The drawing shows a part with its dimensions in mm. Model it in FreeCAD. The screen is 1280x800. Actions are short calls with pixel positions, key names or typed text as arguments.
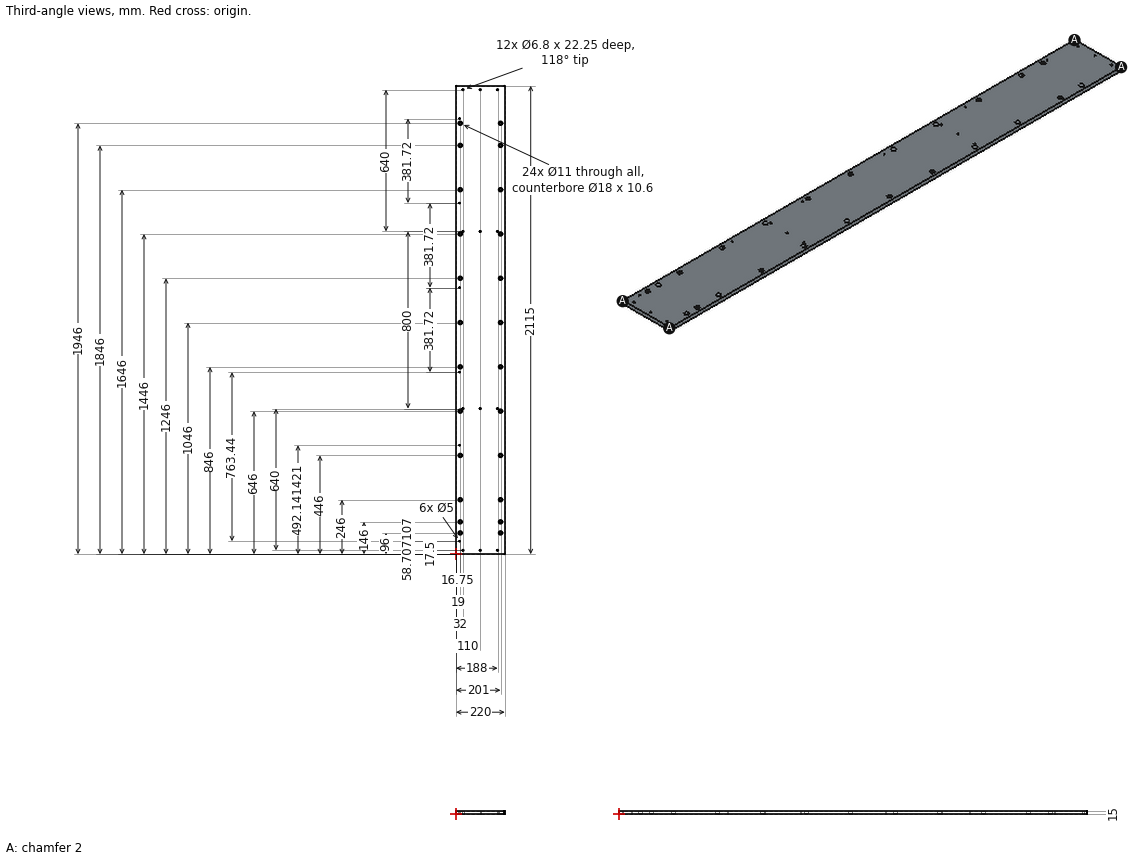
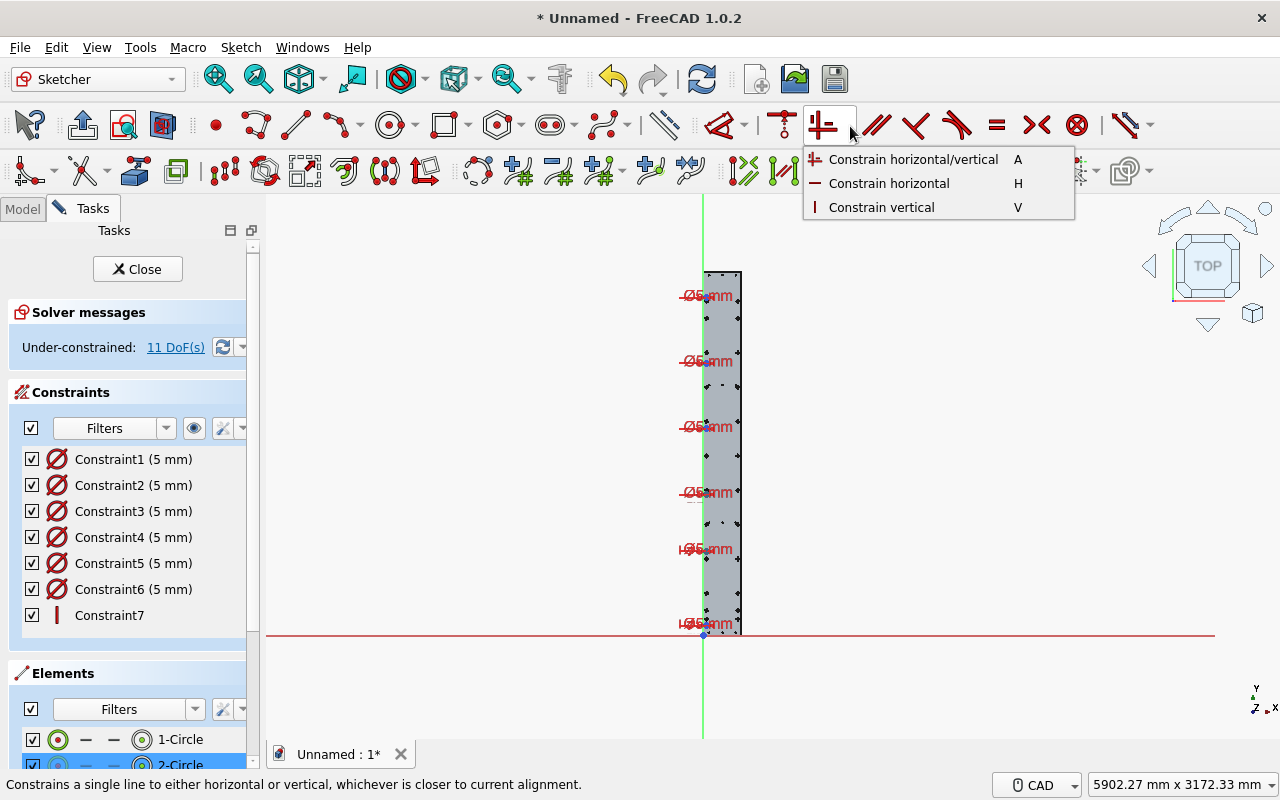
click(939, 207)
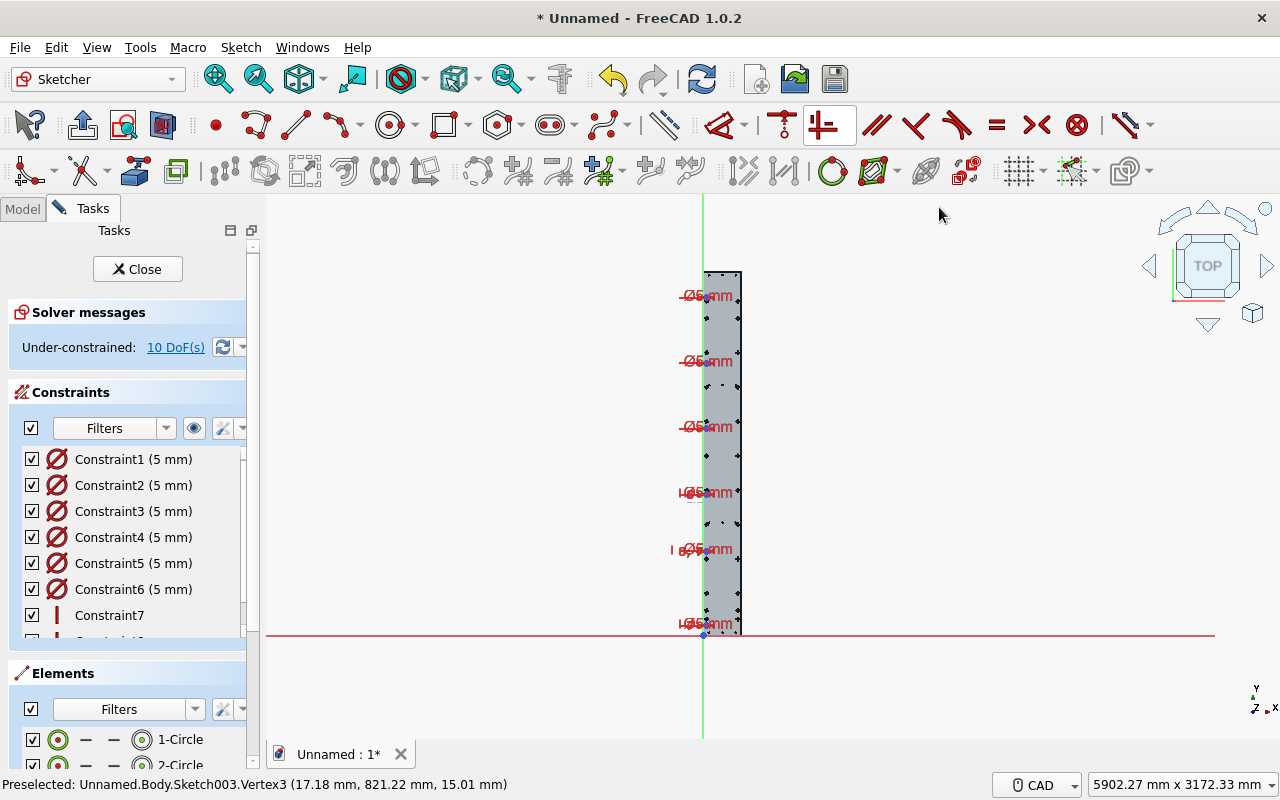
click(706, 495)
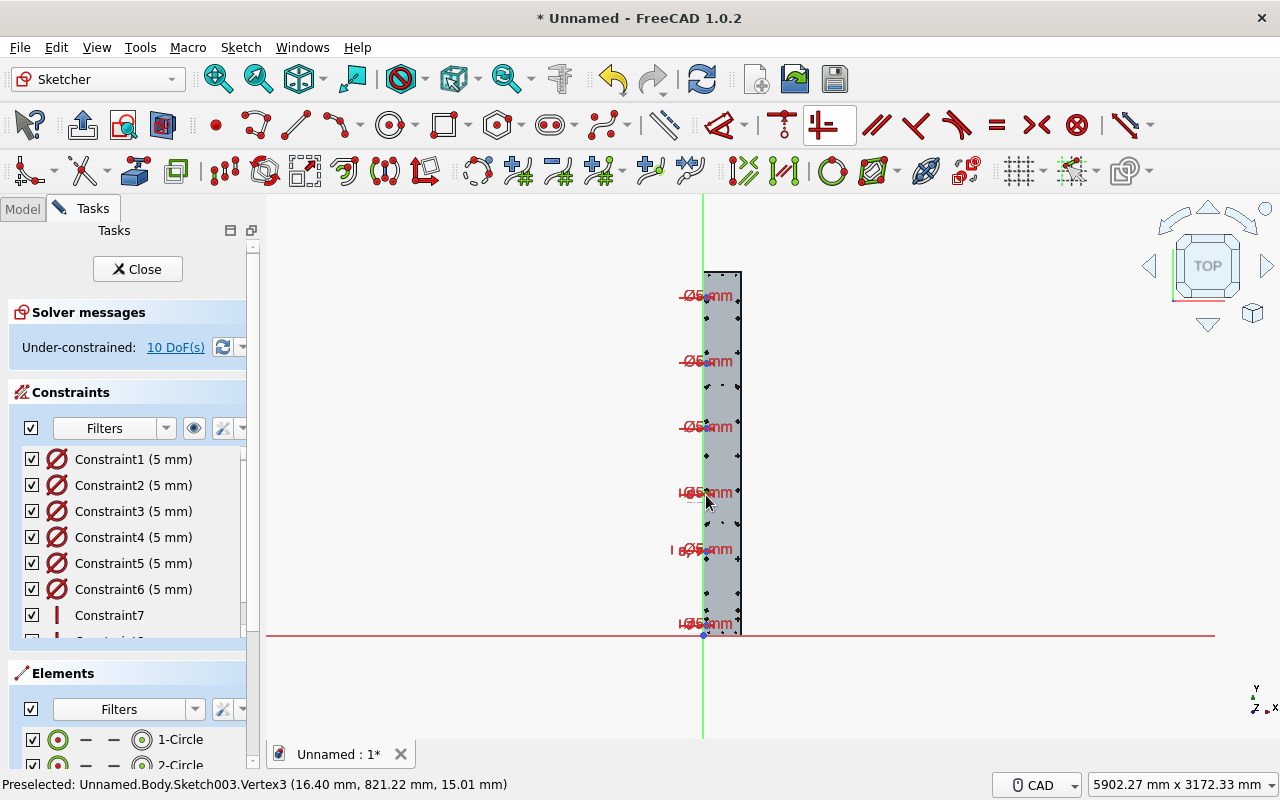
click(706, 429)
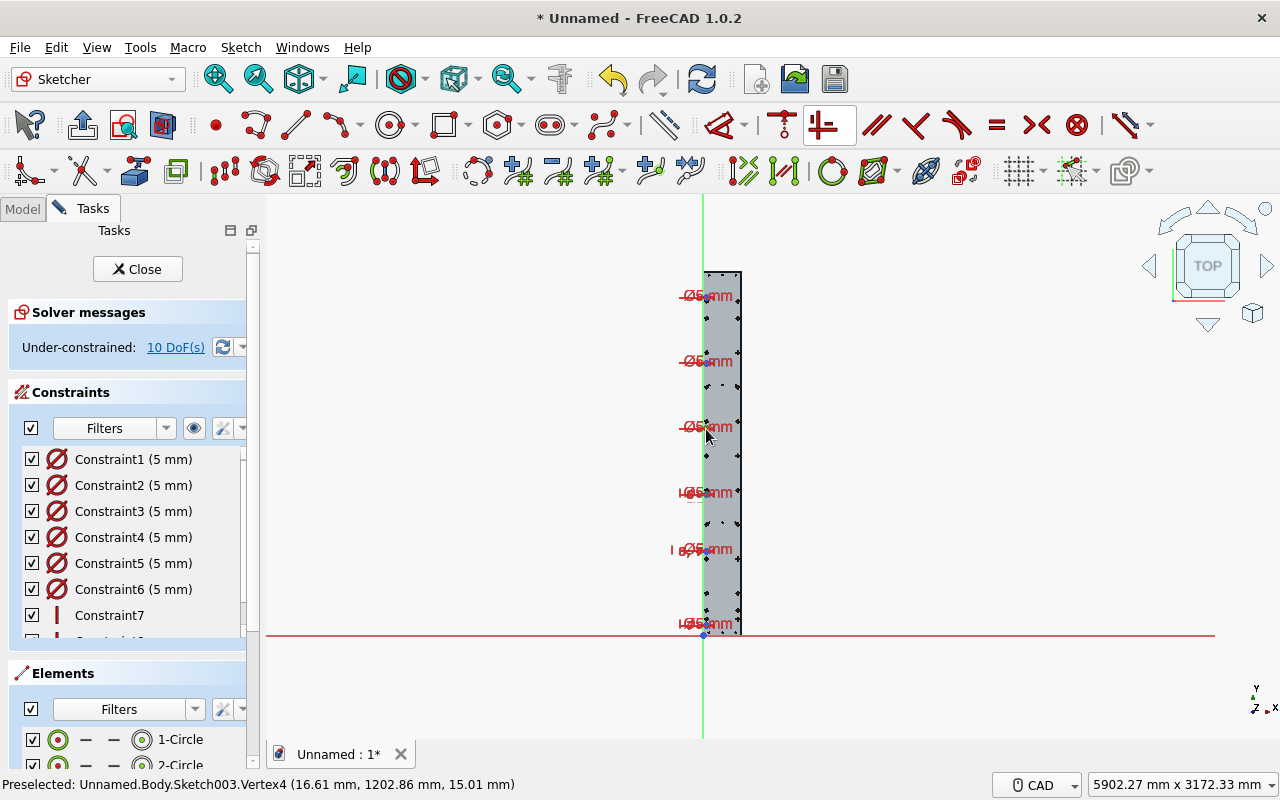
key(v)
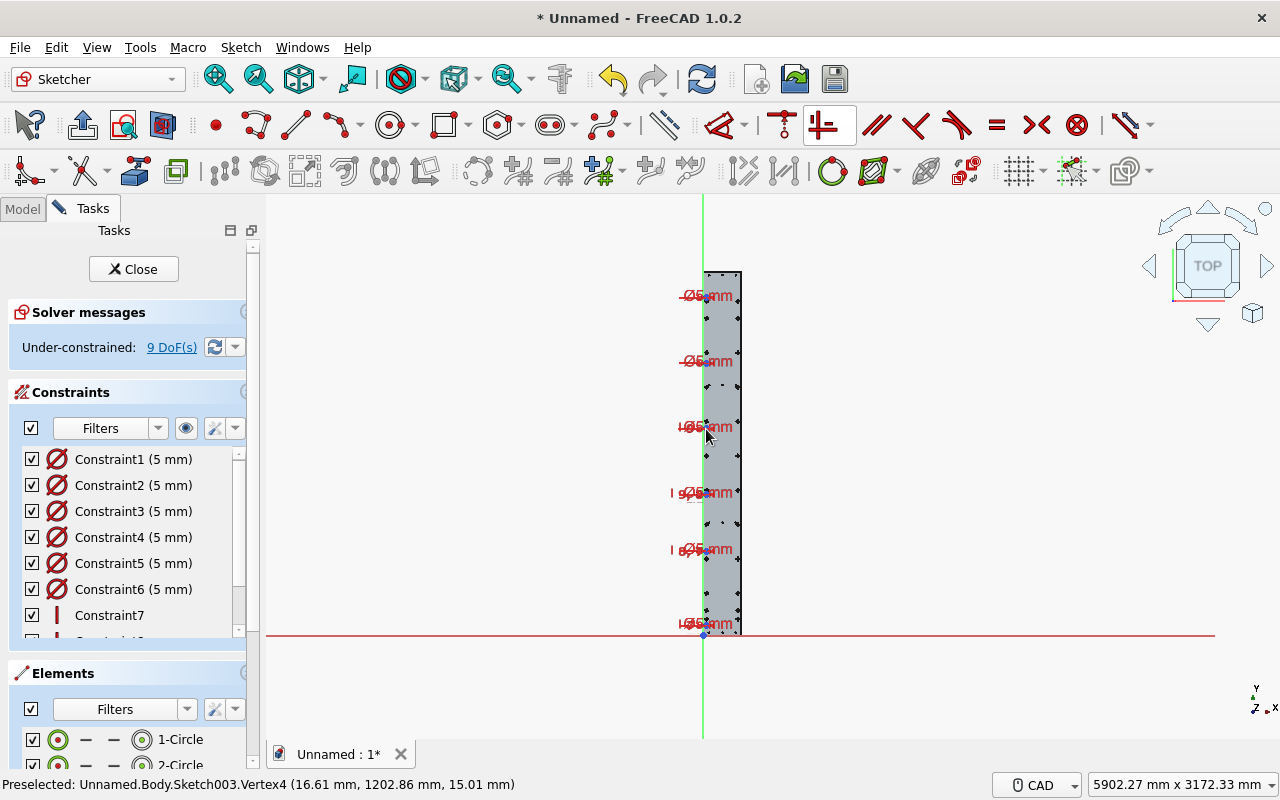
click(706, 429)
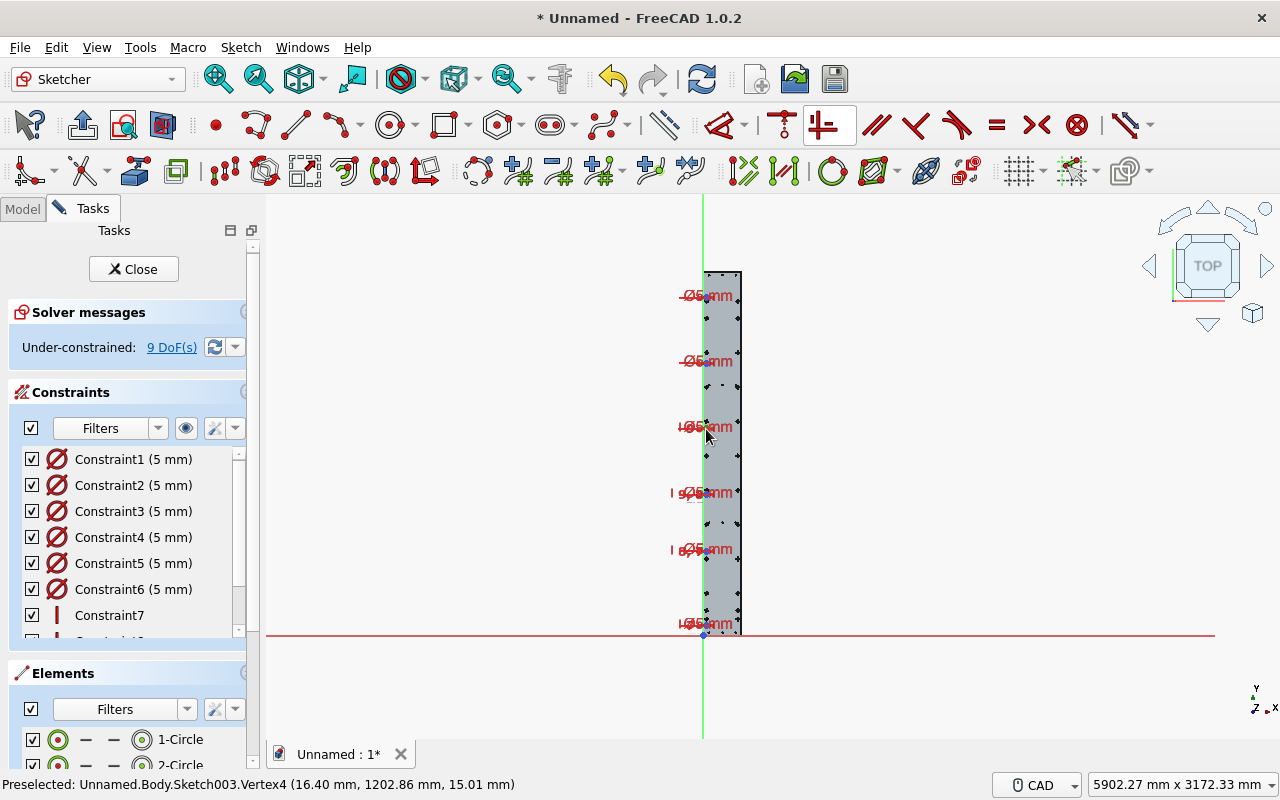
click(706, 363)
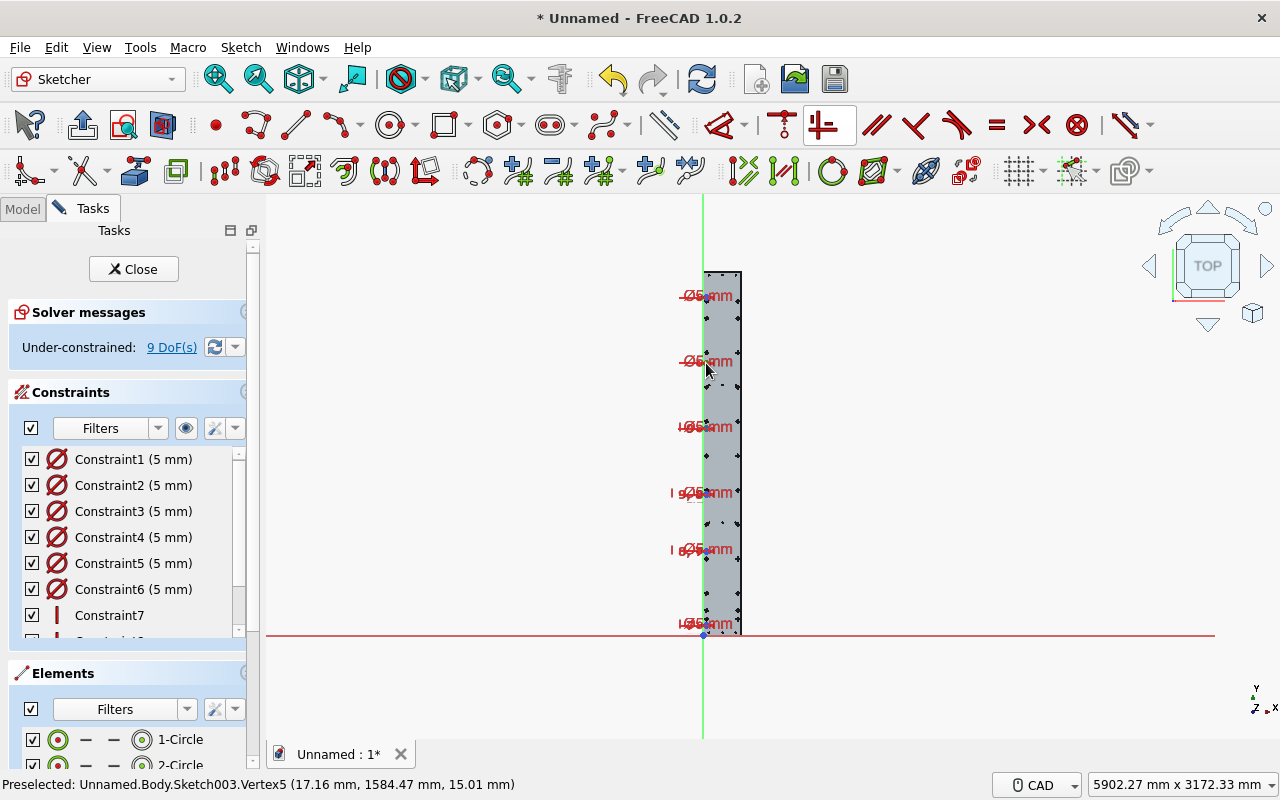
click(850, 126)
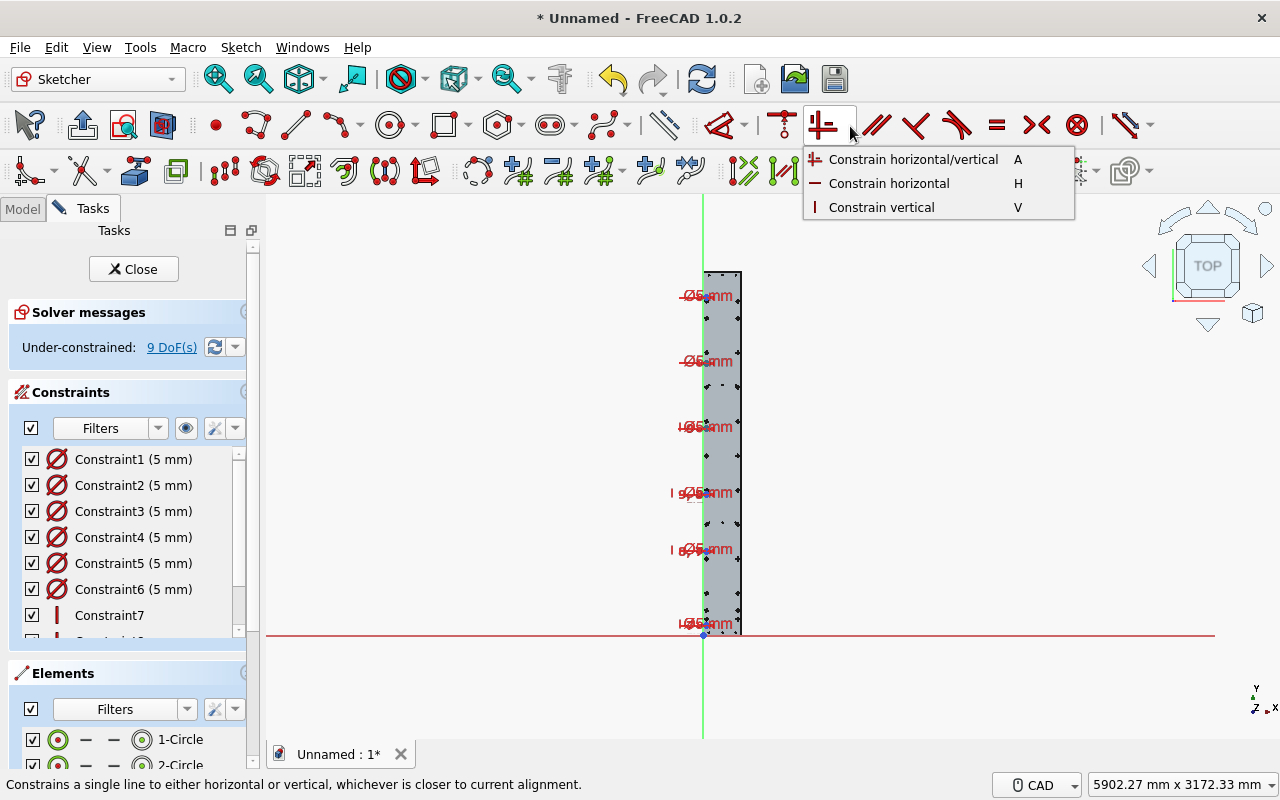
click(939, 207)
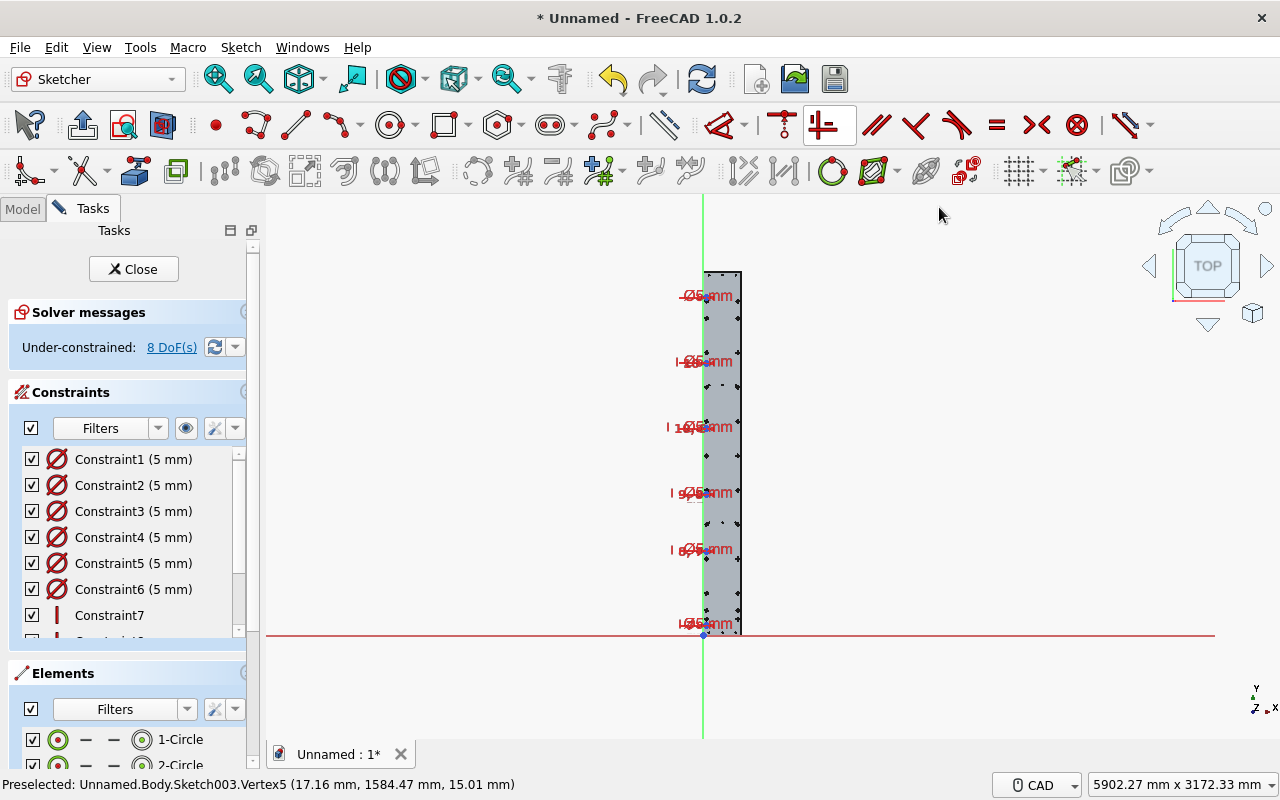
click(706, 363)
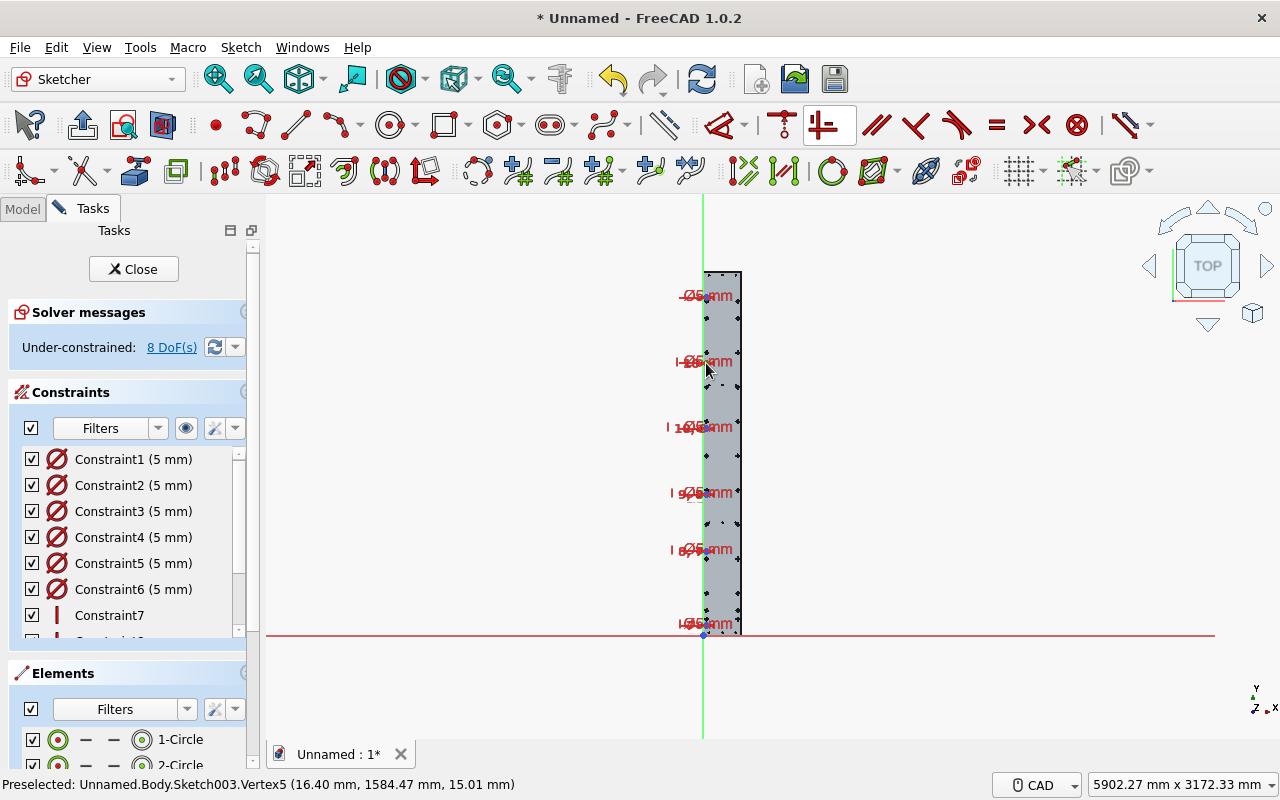
click(706, 298)